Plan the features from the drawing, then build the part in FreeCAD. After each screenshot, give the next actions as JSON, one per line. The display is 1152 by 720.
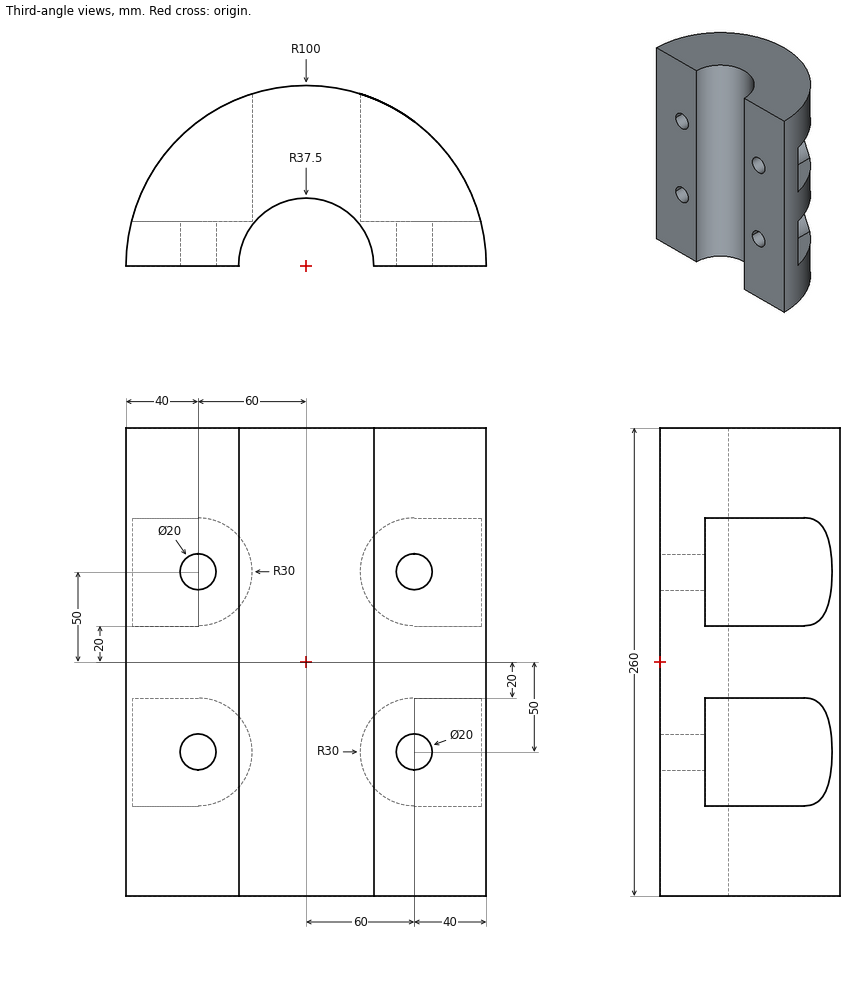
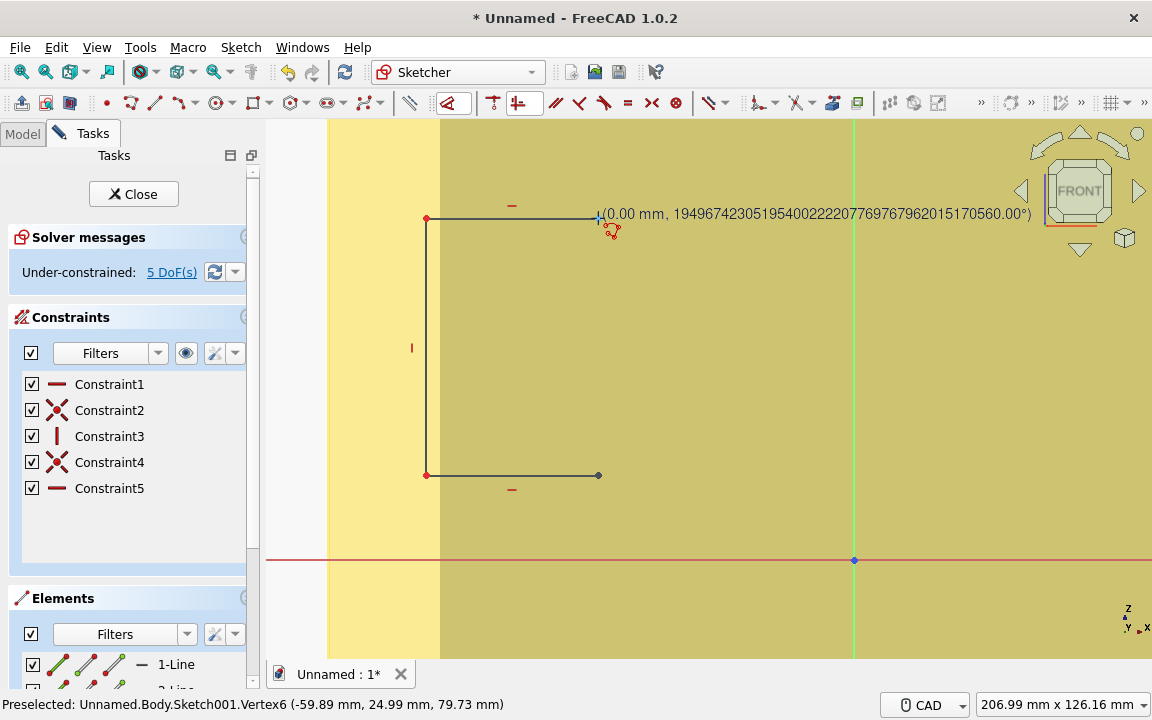
{"action": "left_click", "coordinate": [180, 104]}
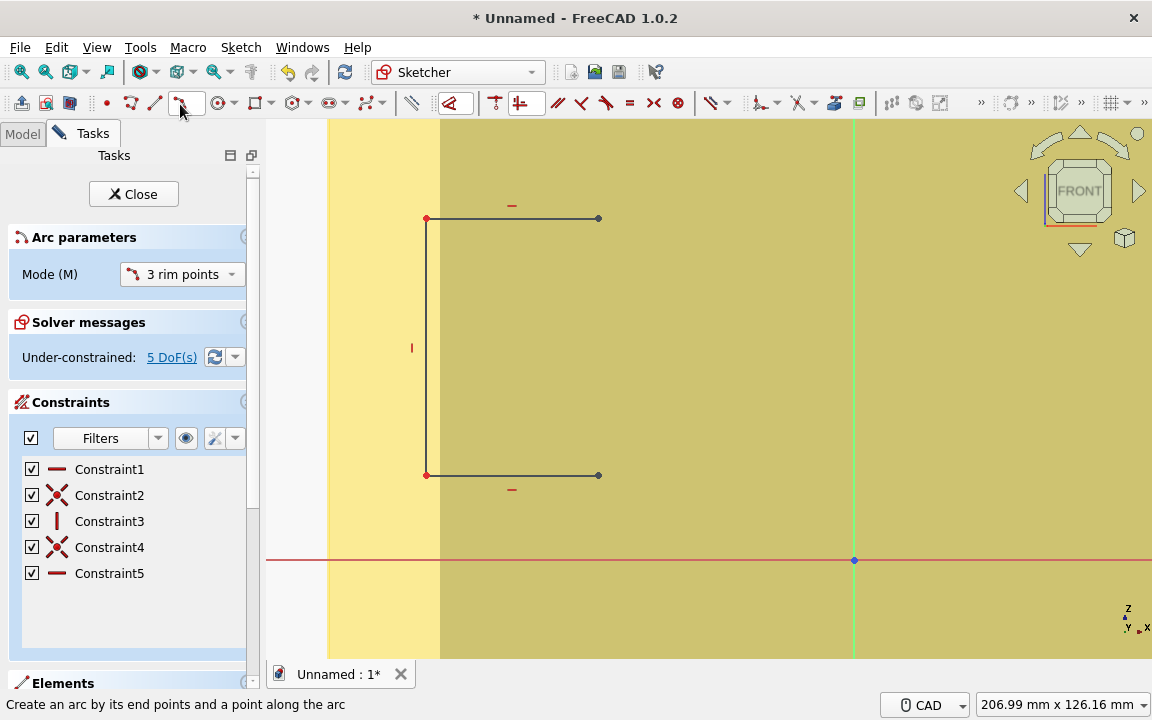
{"action": "left_click", "coordinate": [598, 219]}
{"action": "left_click", "coordinate": [598, 476]}
{"action": "left_click", "coordinate": [726, 346]}
{"action": "key", "text": "Escape"}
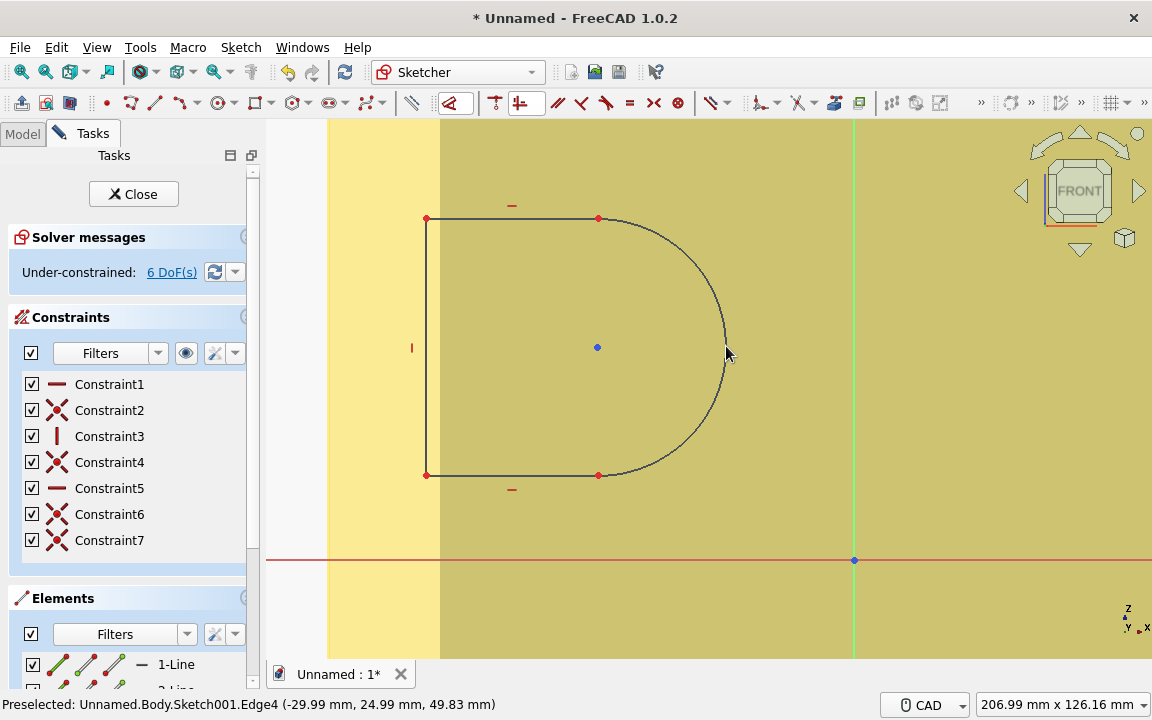
{"action": "left_click", "coordinate": [546, 476]}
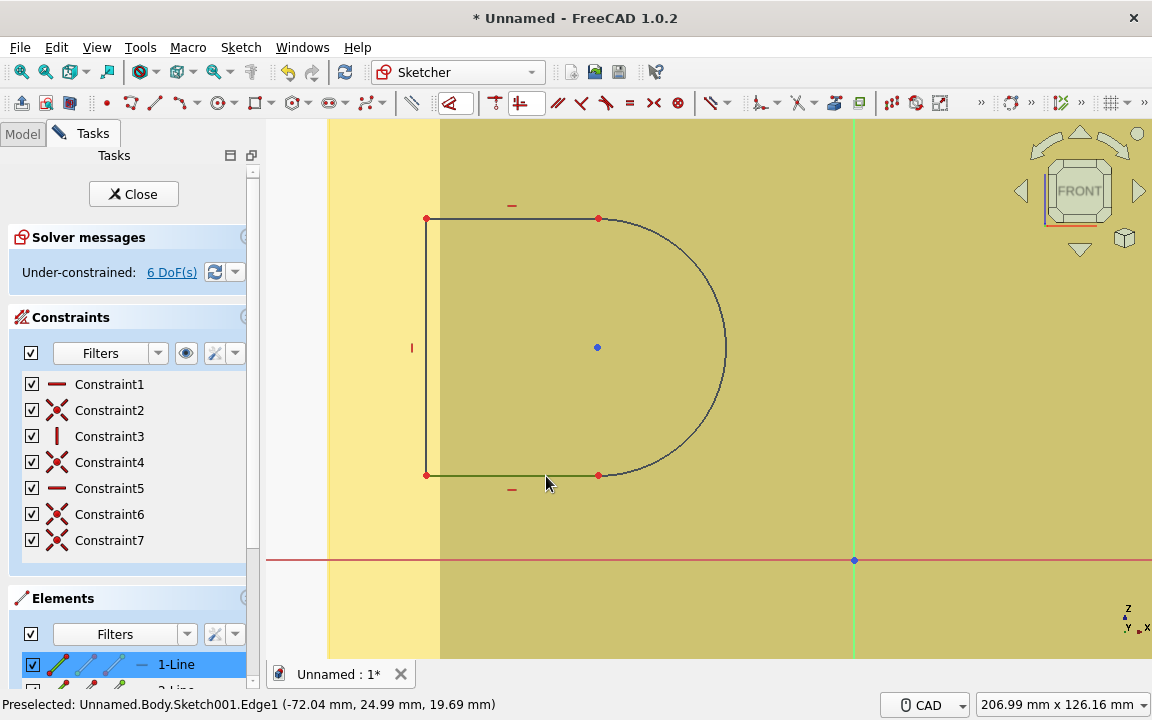
{"action": "left_click", "coordinate": [702, 423]}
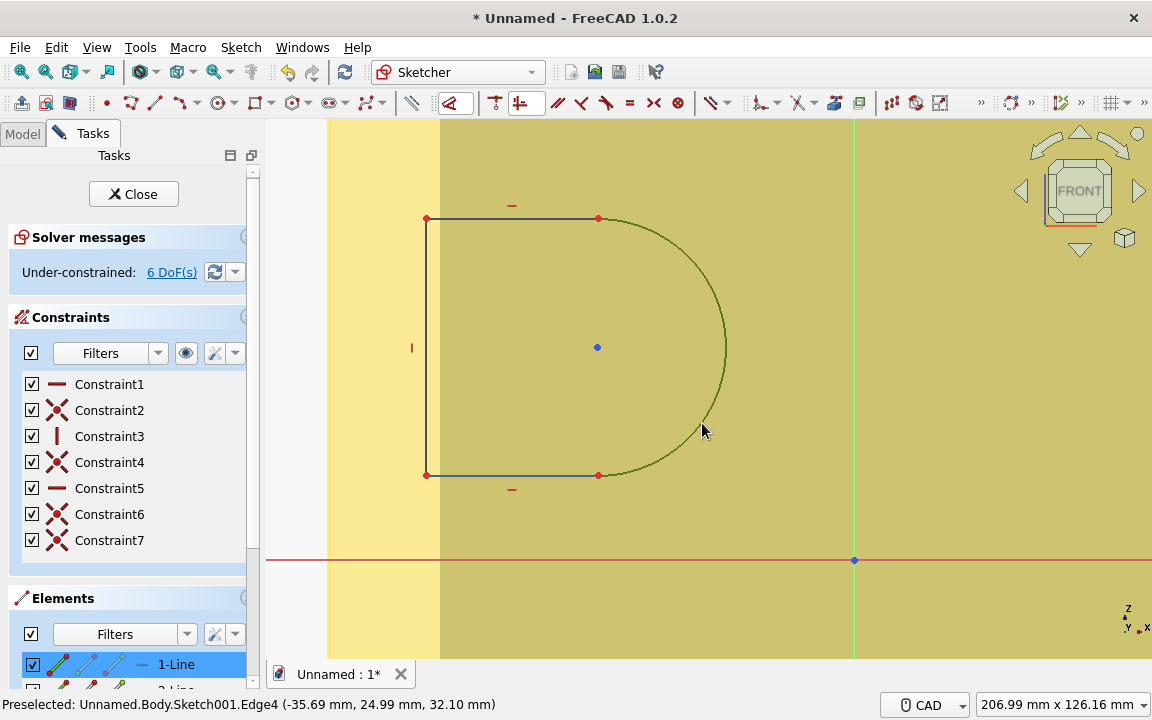
{"action": "left_click", "coordinate": [606, 104]}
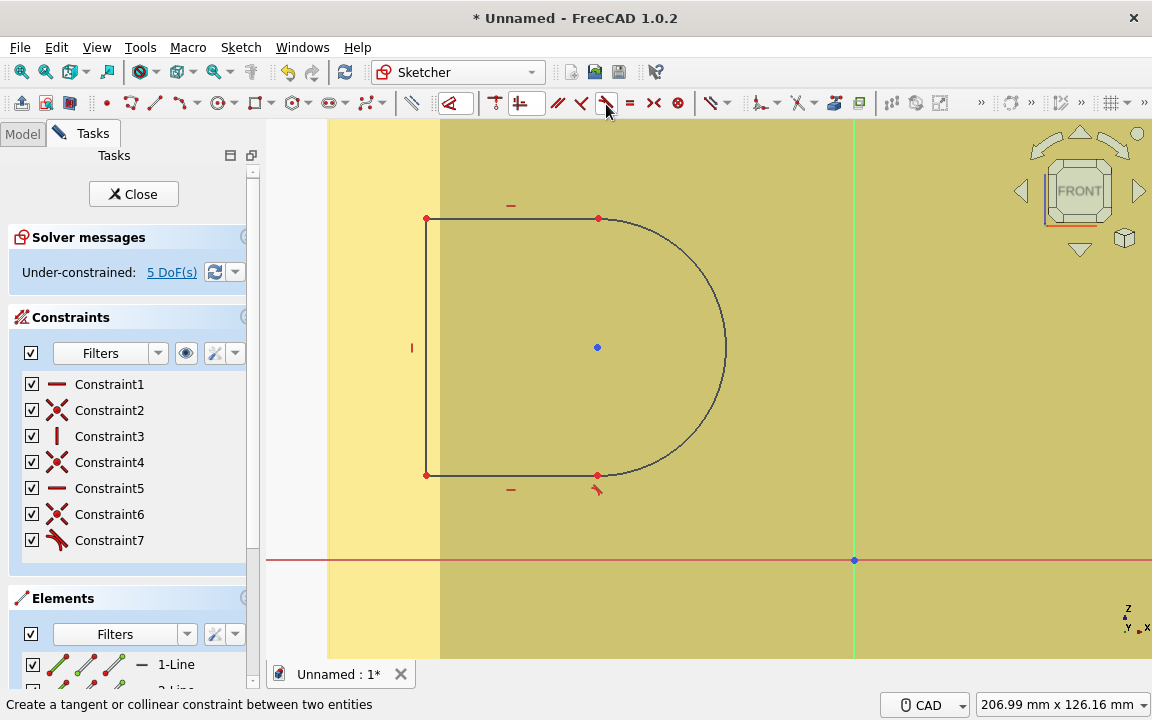
{"action": "left_click", "coordinate": [478, 219]}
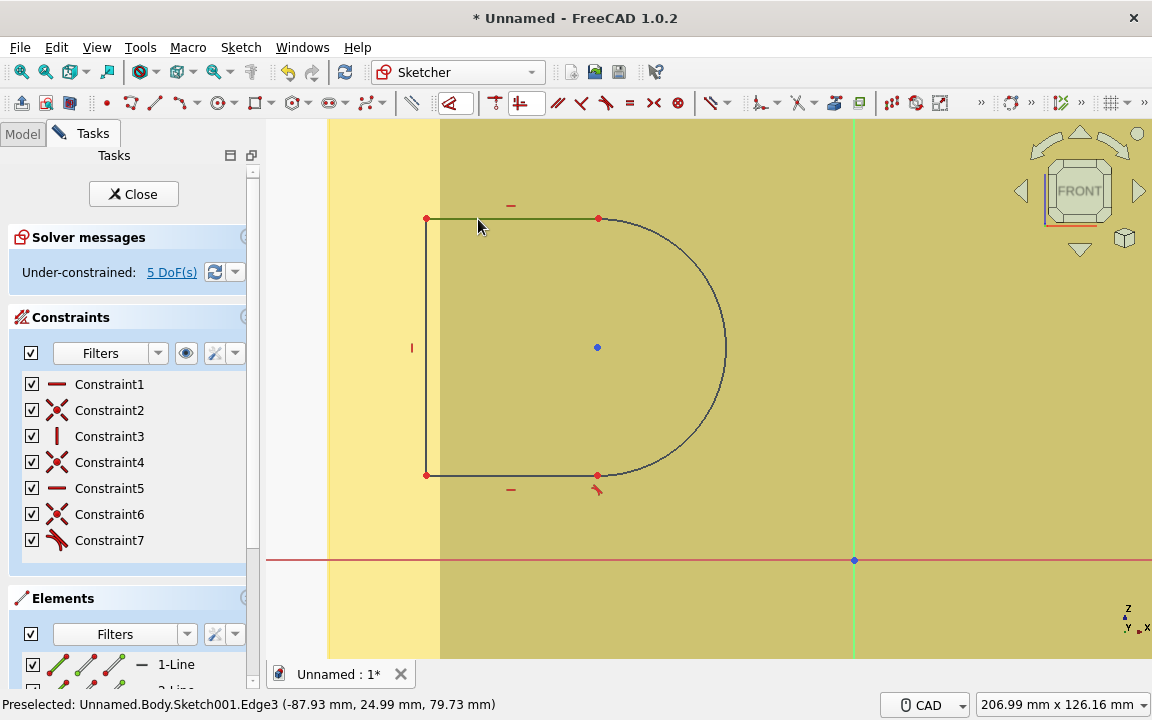
{"action": "left_click", "coordinate": [701, 423]}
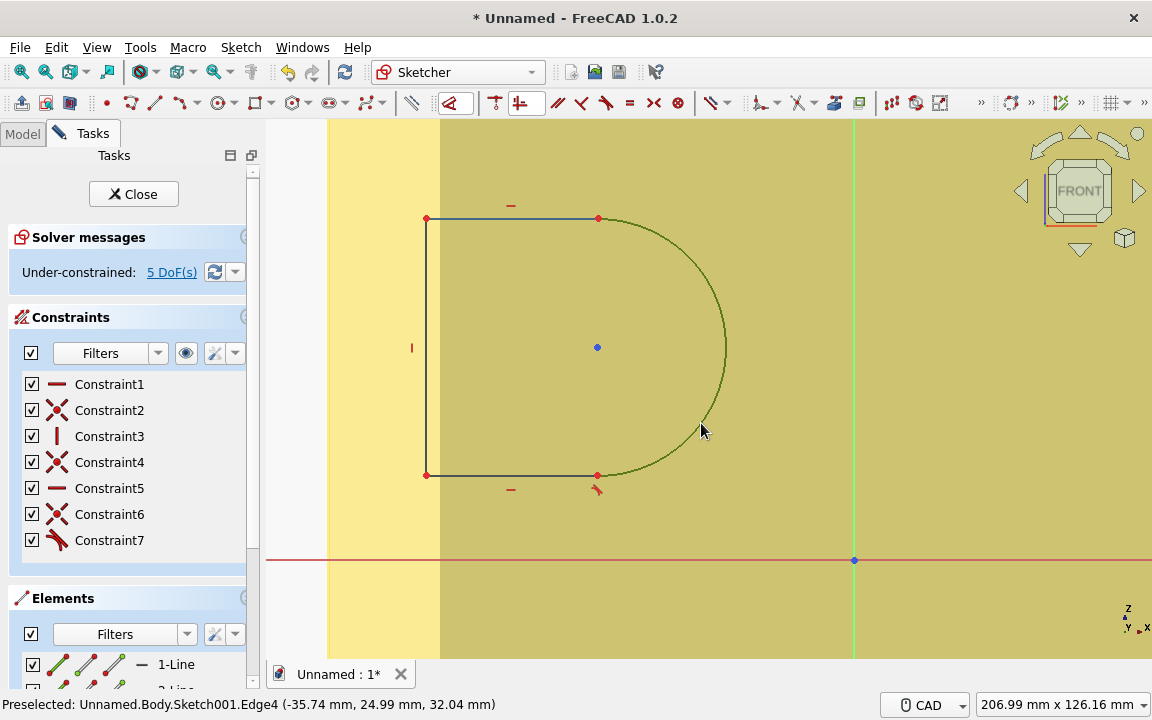
{"action": "left_click", "coordinate": [606, 104]}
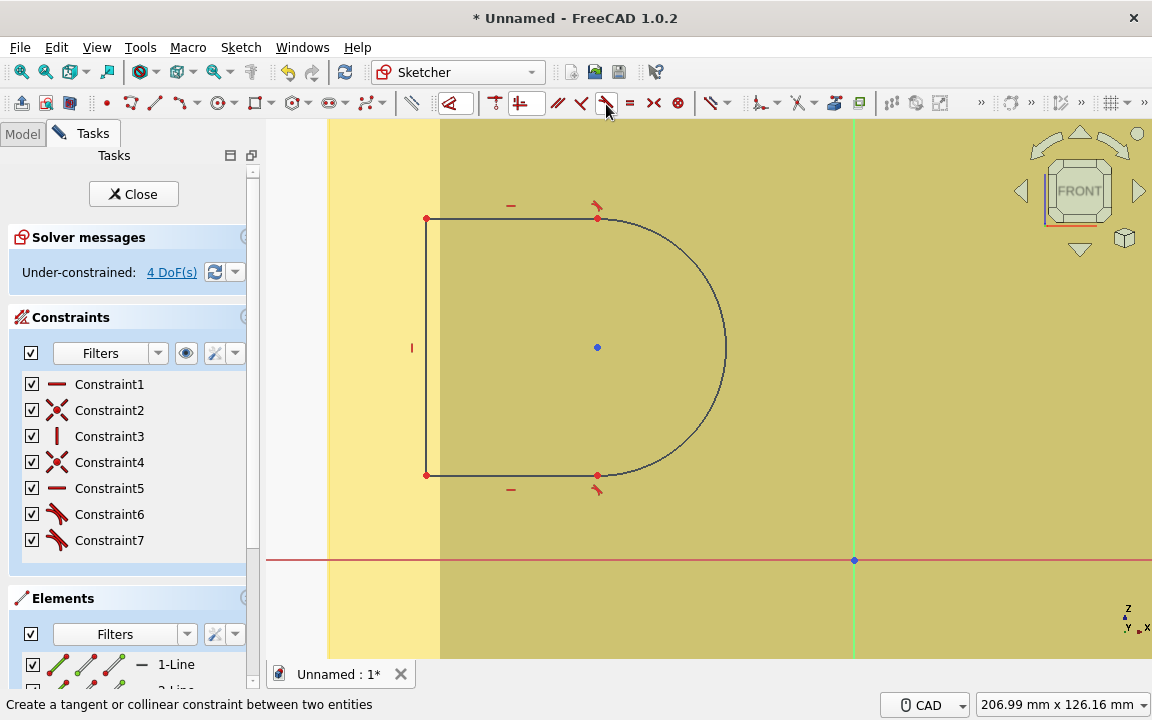
{"action": "left_click", "coordinate": [702, 423]}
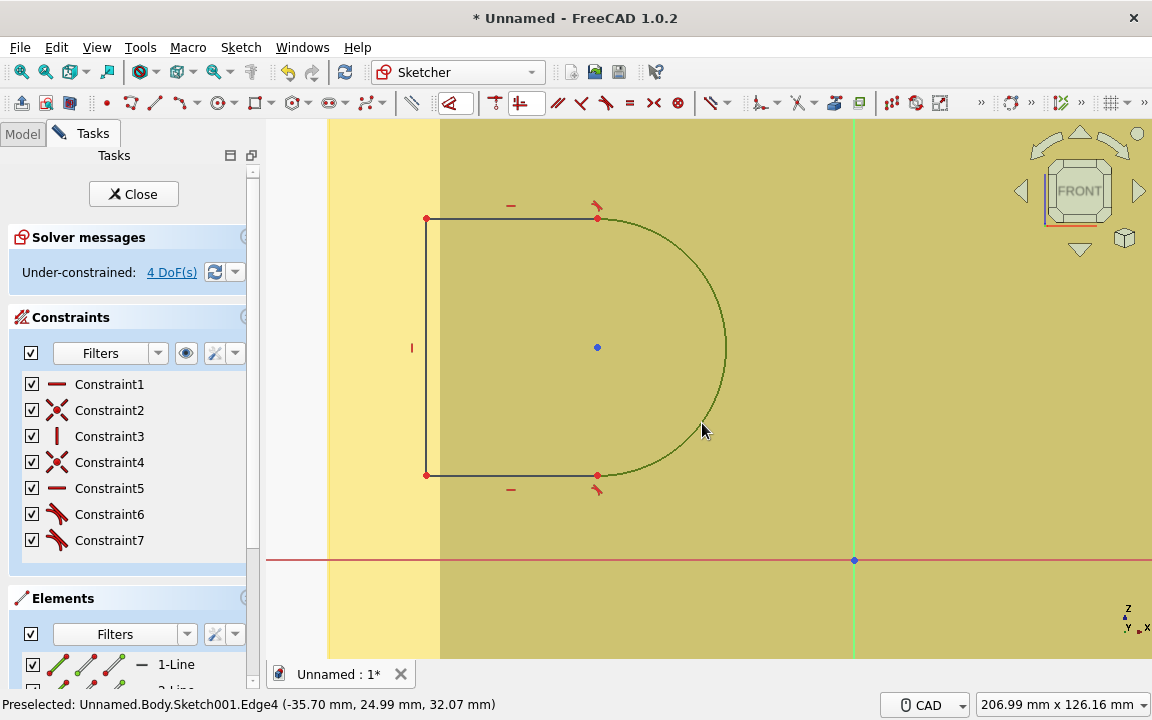
{"action": "key", "text": "k r"}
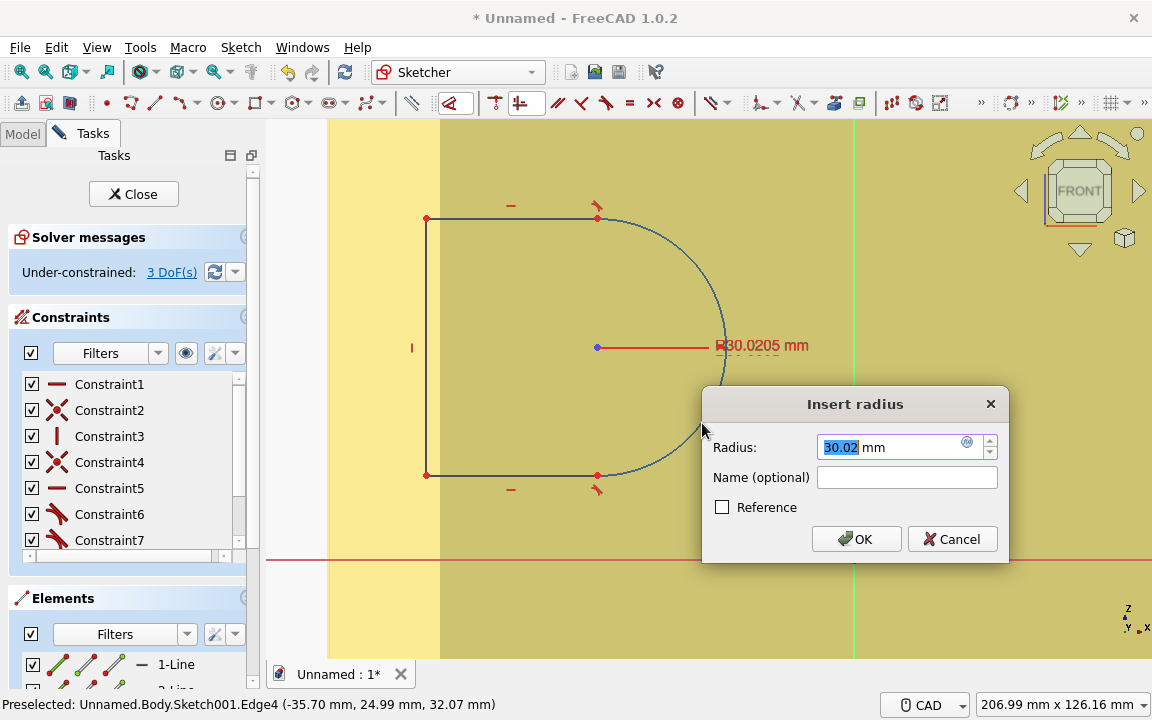
{"action": "type", "text": "30"}
{"action": "key", "text": "Return"}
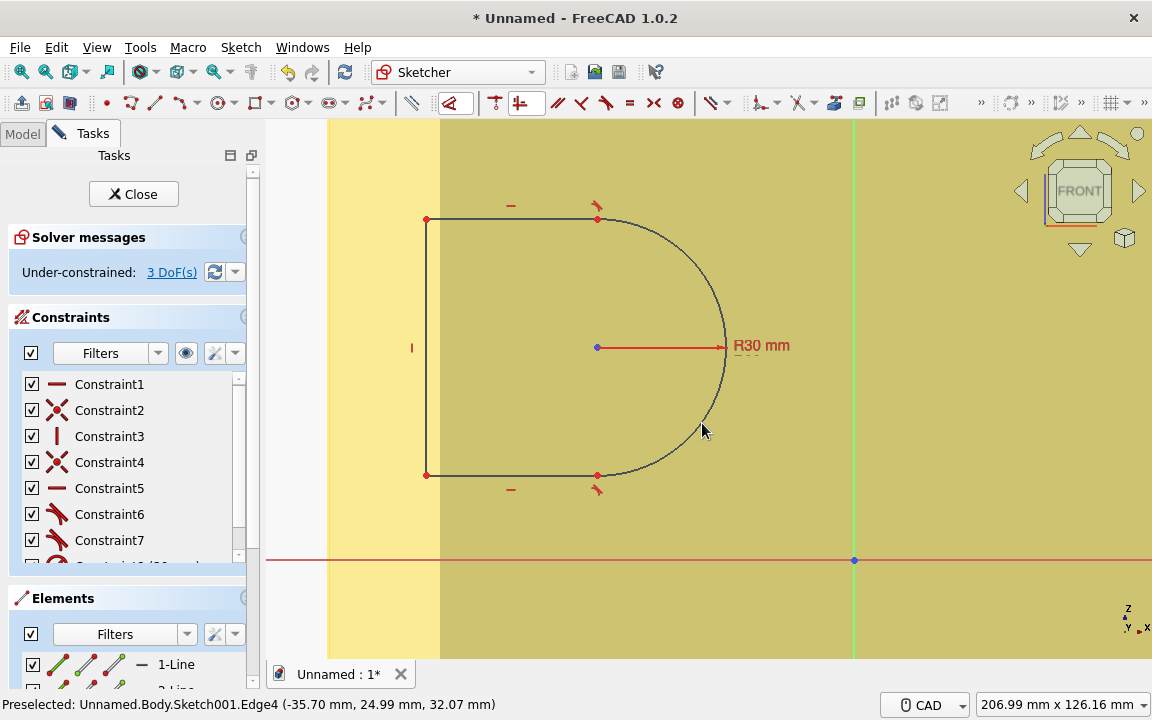
{"action": "left_click", "coordinate": [546, 476]}